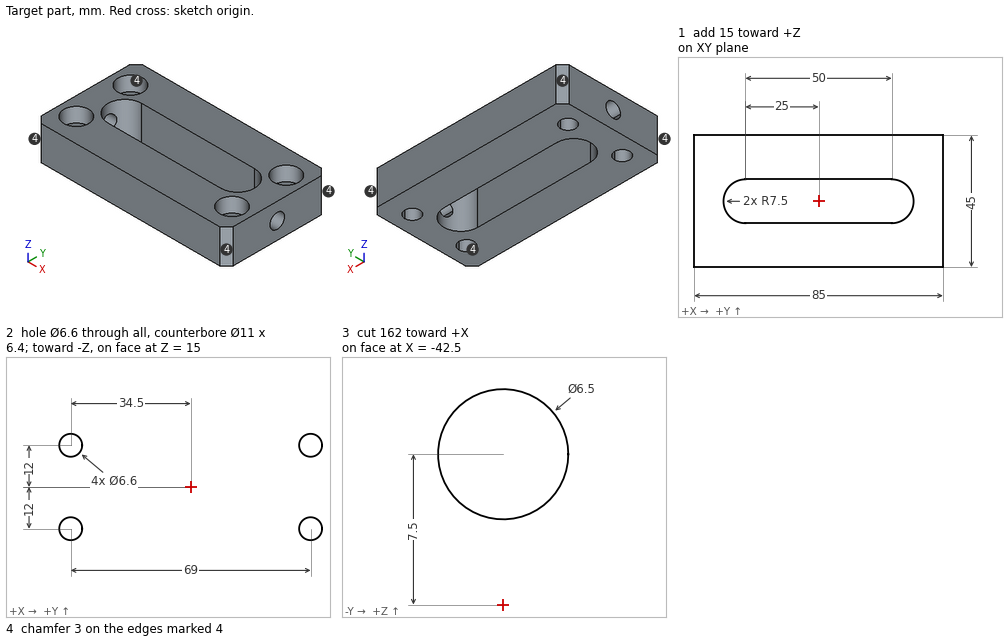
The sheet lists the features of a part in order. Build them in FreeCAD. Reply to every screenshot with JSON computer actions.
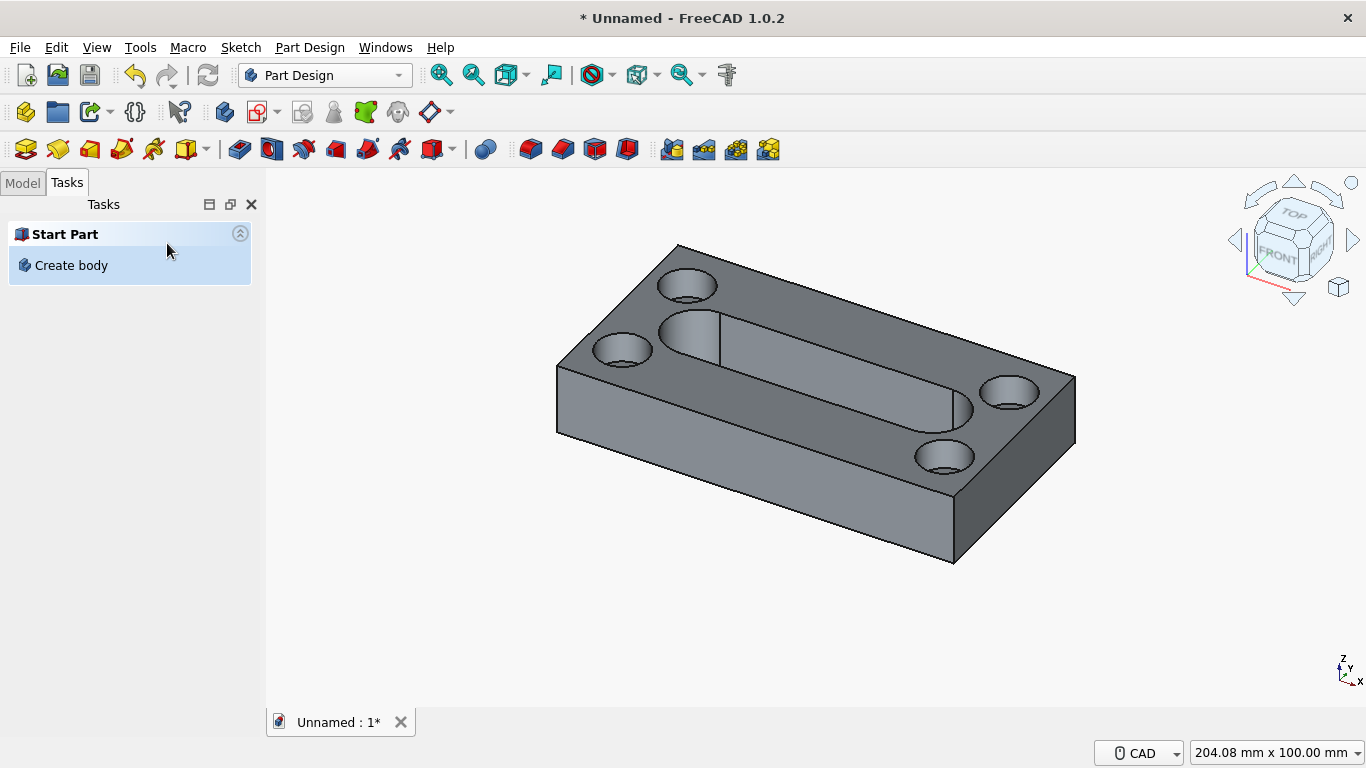
{"action": "key", "text": "6"}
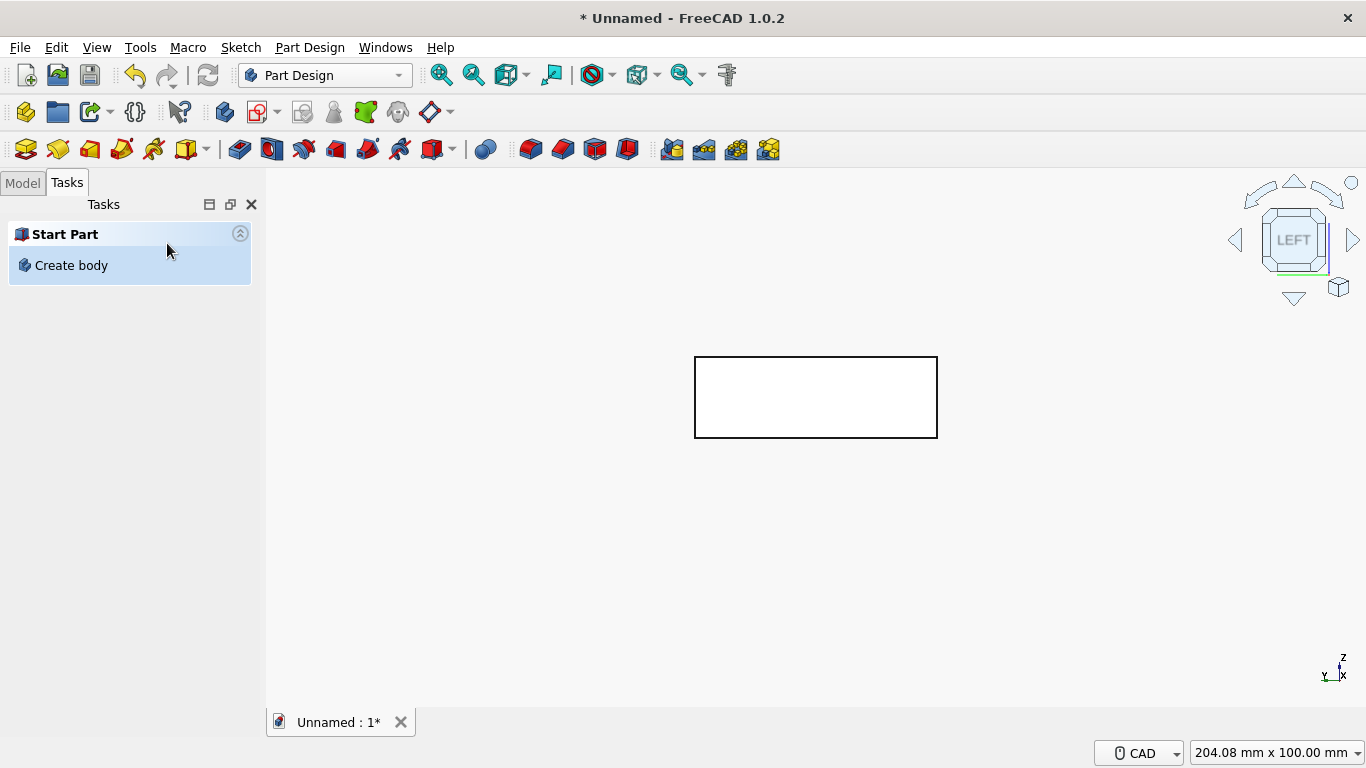
{"action": "key", "text": "v f"}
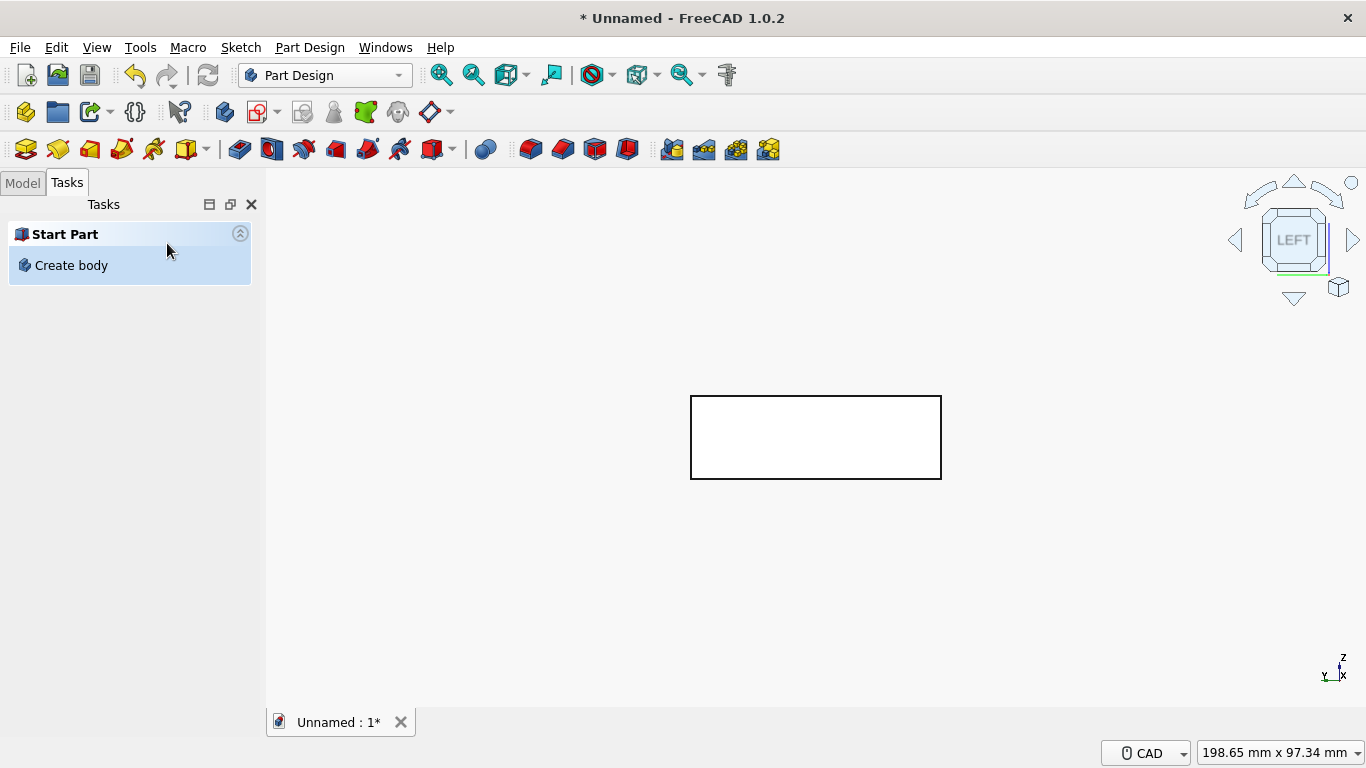
{"action": "left_click", "coordinate": [745, 436]}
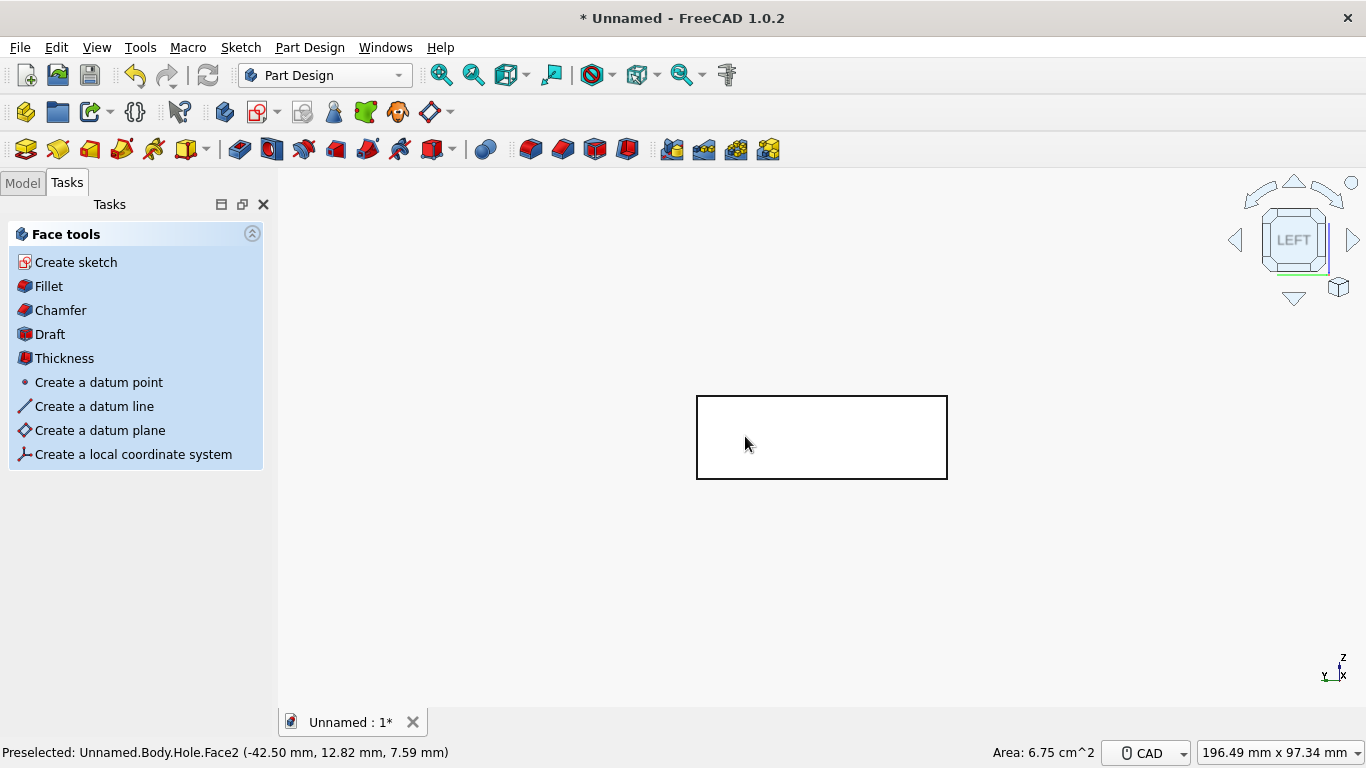
{"action": "left_click", "coordinate": [258, 112]}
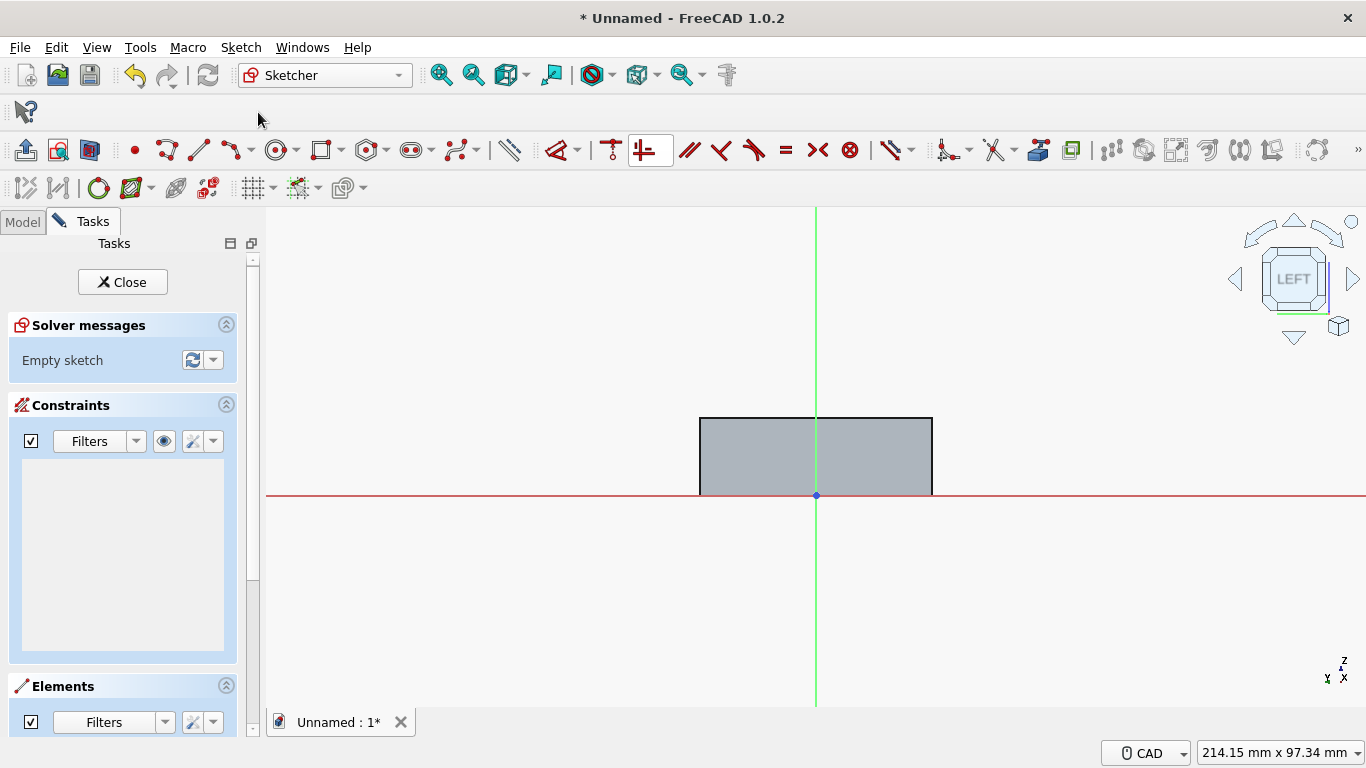
{"action": "scroll", "coordinate": [830, 470], "scroll_direction": "up", "scroll_amount": 9}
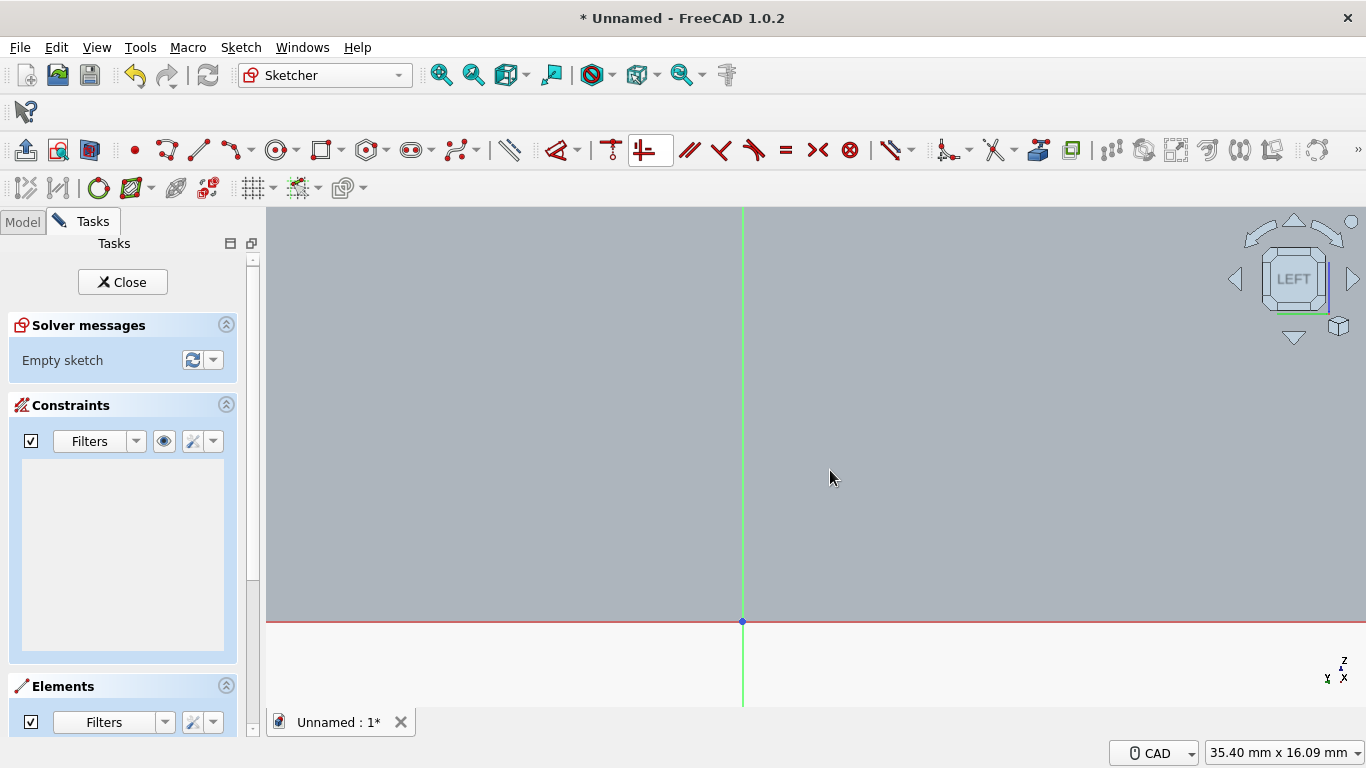
{"action": "left_click", "coordinate": [276, 150]}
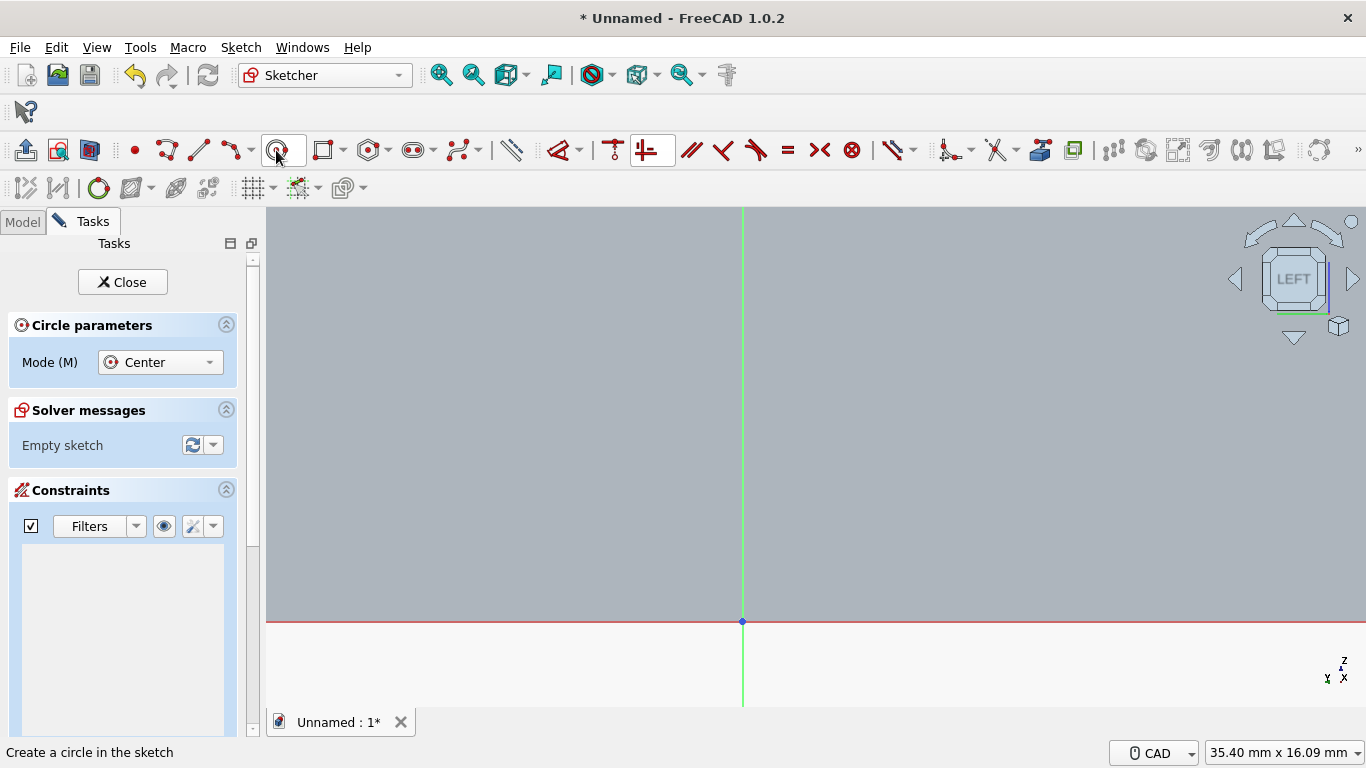
{"action": "left_click", "coordinate": [743, 389]}
{"action": "left_click", "coordinate": [814, 317]}
{"action": "key", "text": "Escape"}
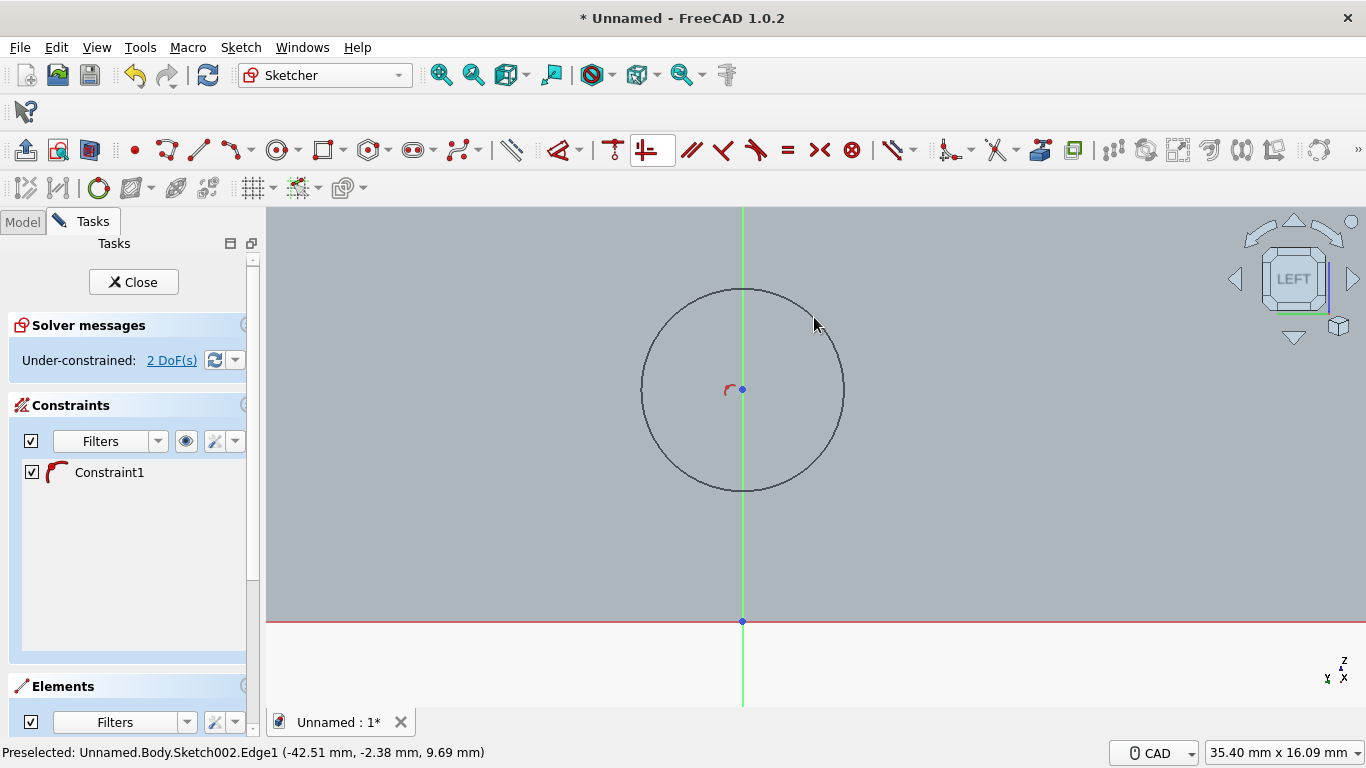
{"action": "left_click", "coordinate": [558, 150]}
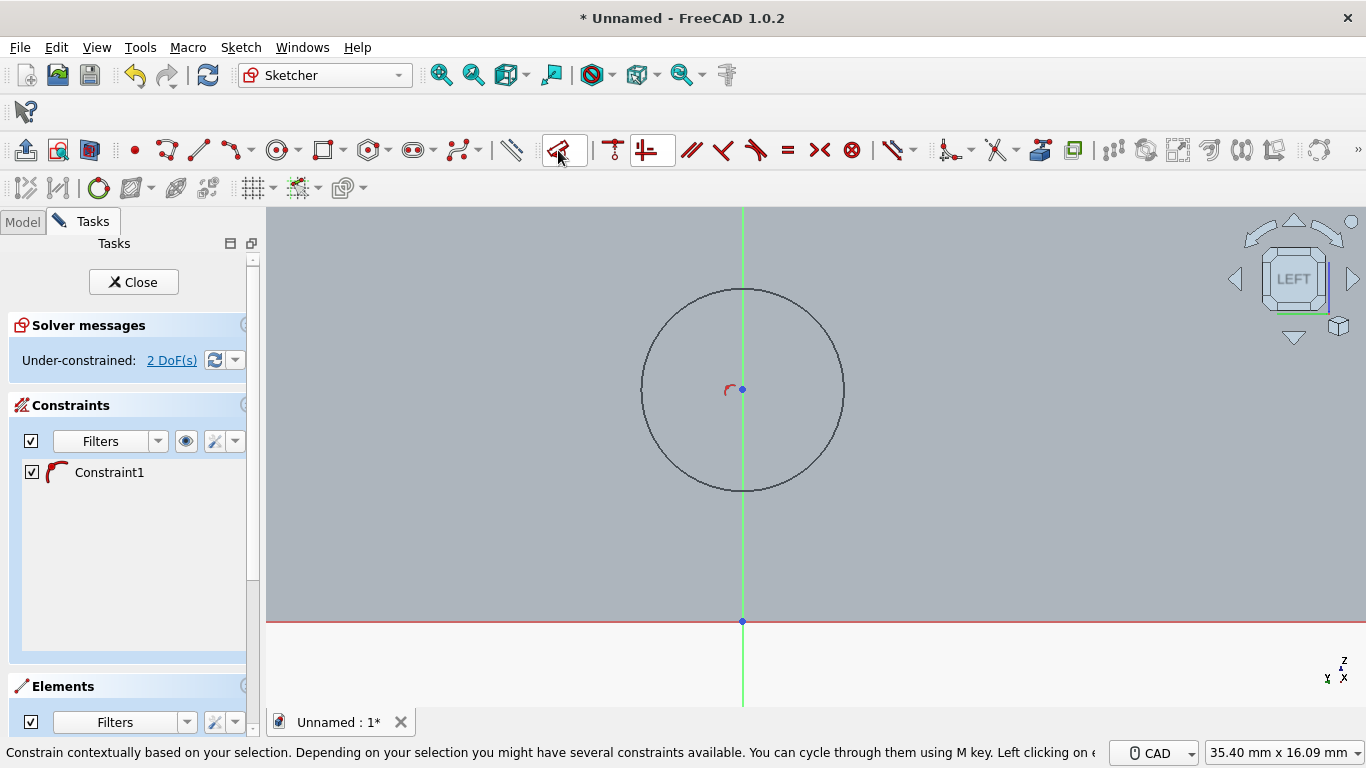
{"action": "left_click", "coordinate": [814, 318]}
{"action": "left_click", "coordinate": [837, 295]}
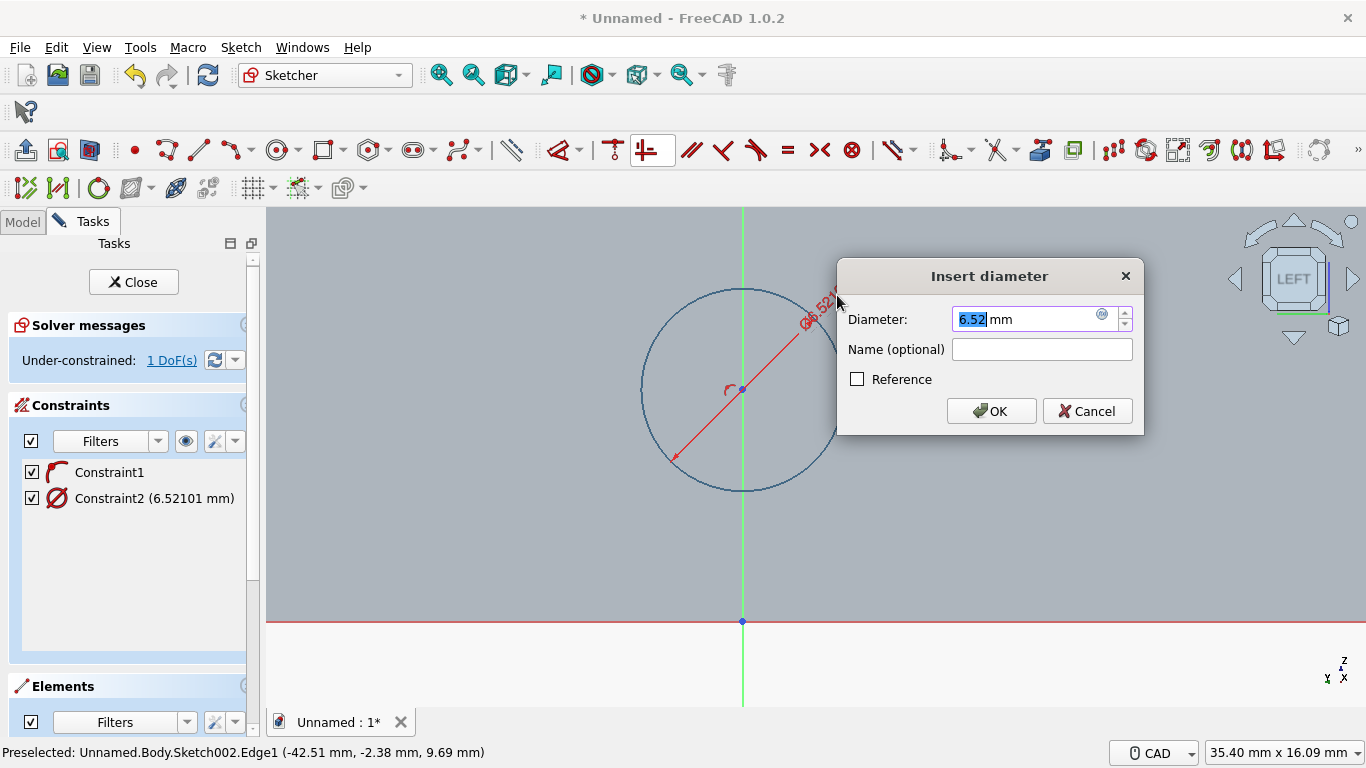
{"action": "type", "text": "6.5"}
{"action": "key", "text": "Return"}